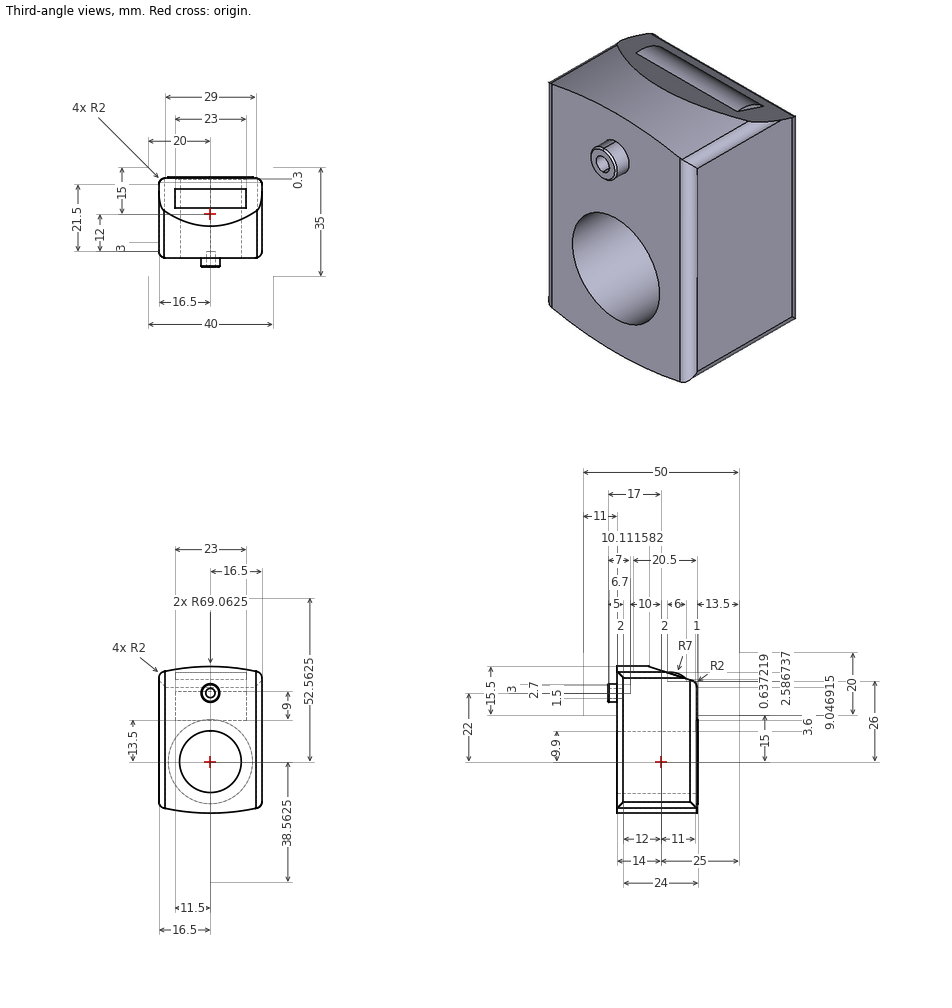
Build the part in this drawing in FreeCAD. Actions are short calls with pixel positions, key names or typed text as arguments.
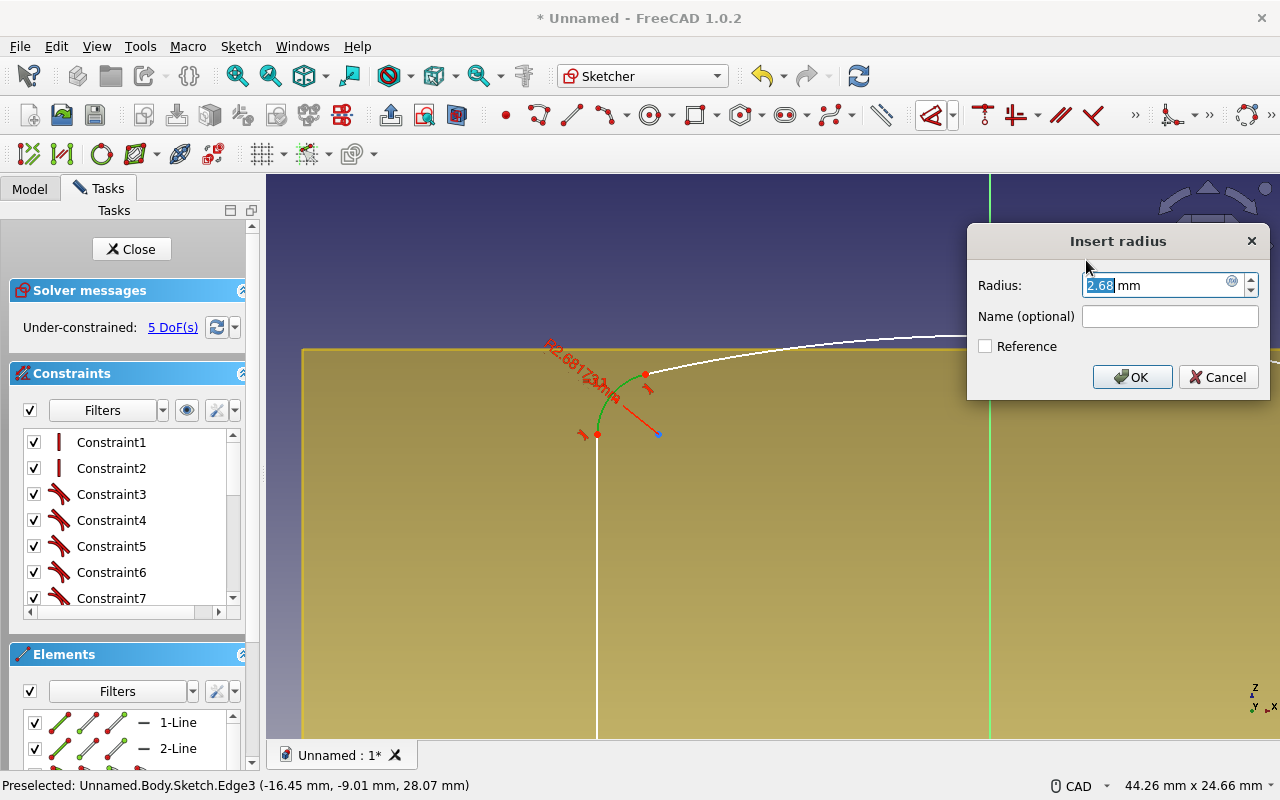
text(2)
key(Return)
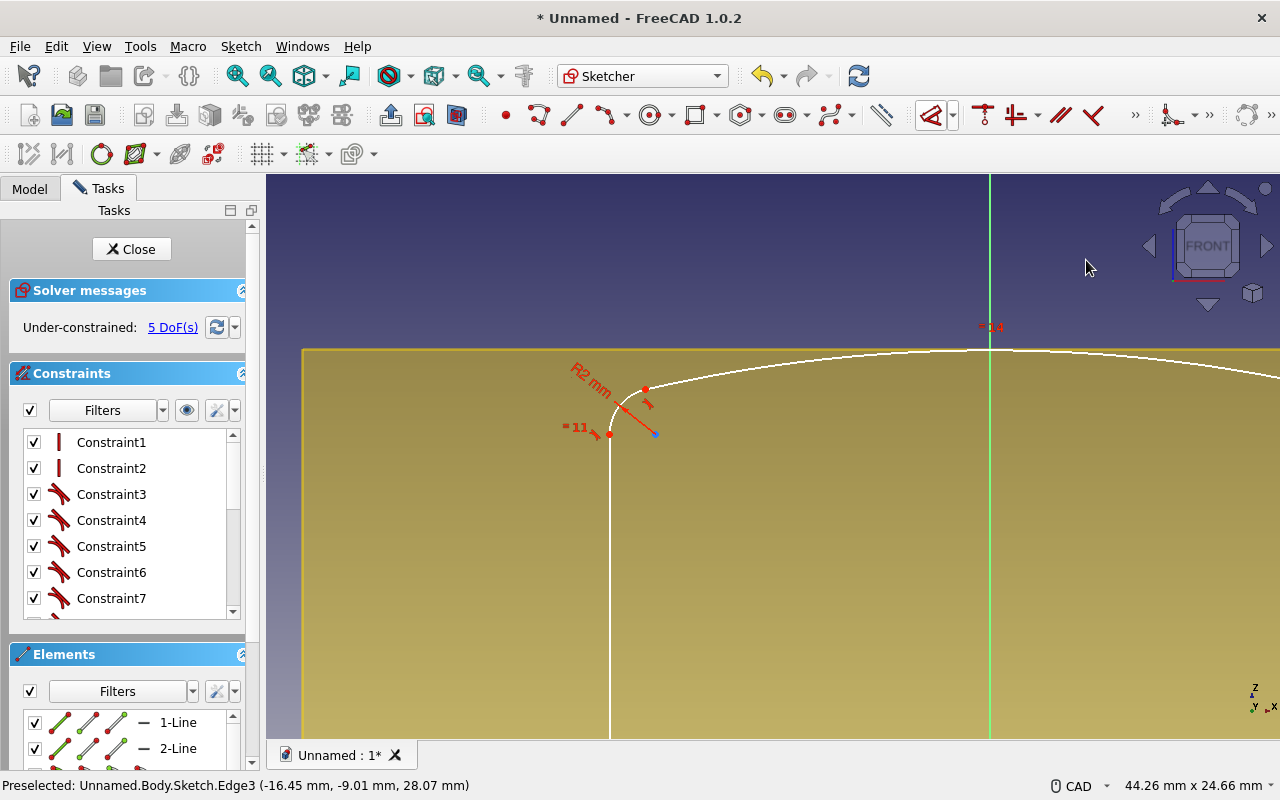
click(851, 357)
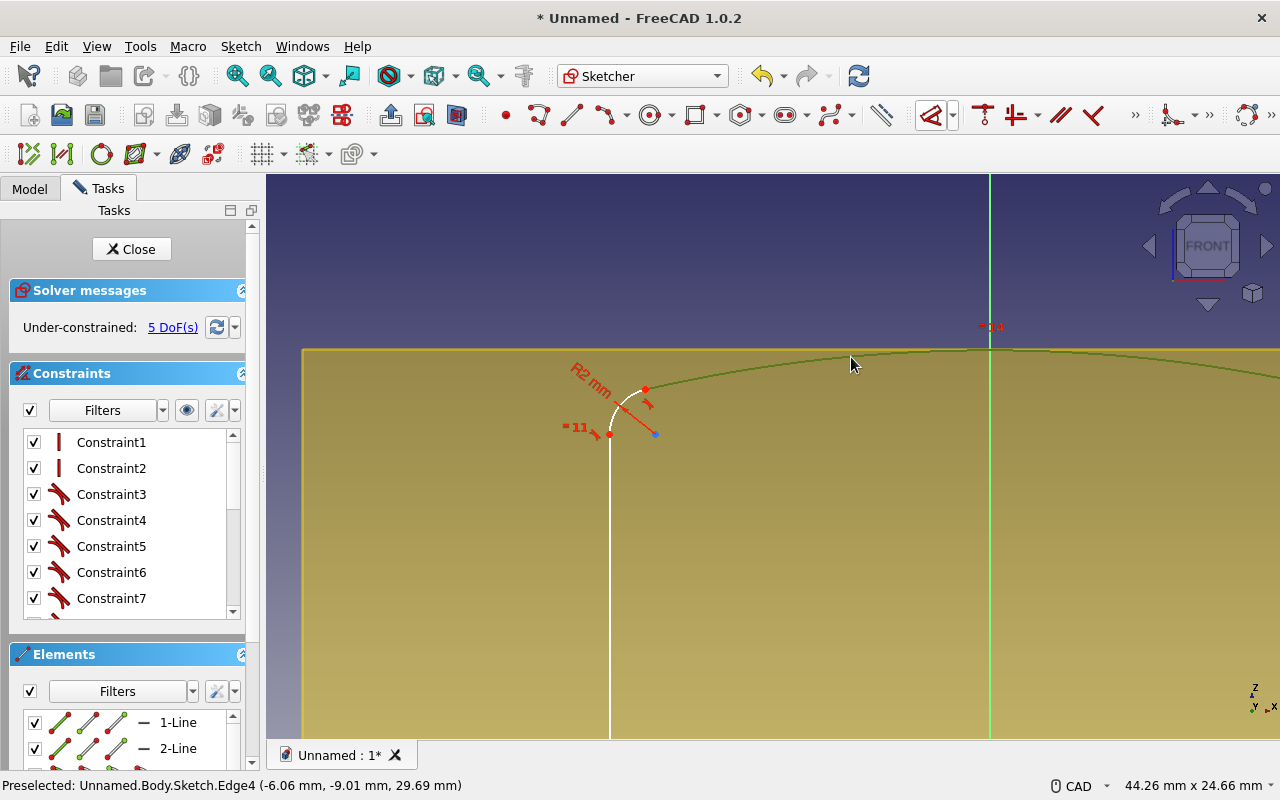
click(952, 116)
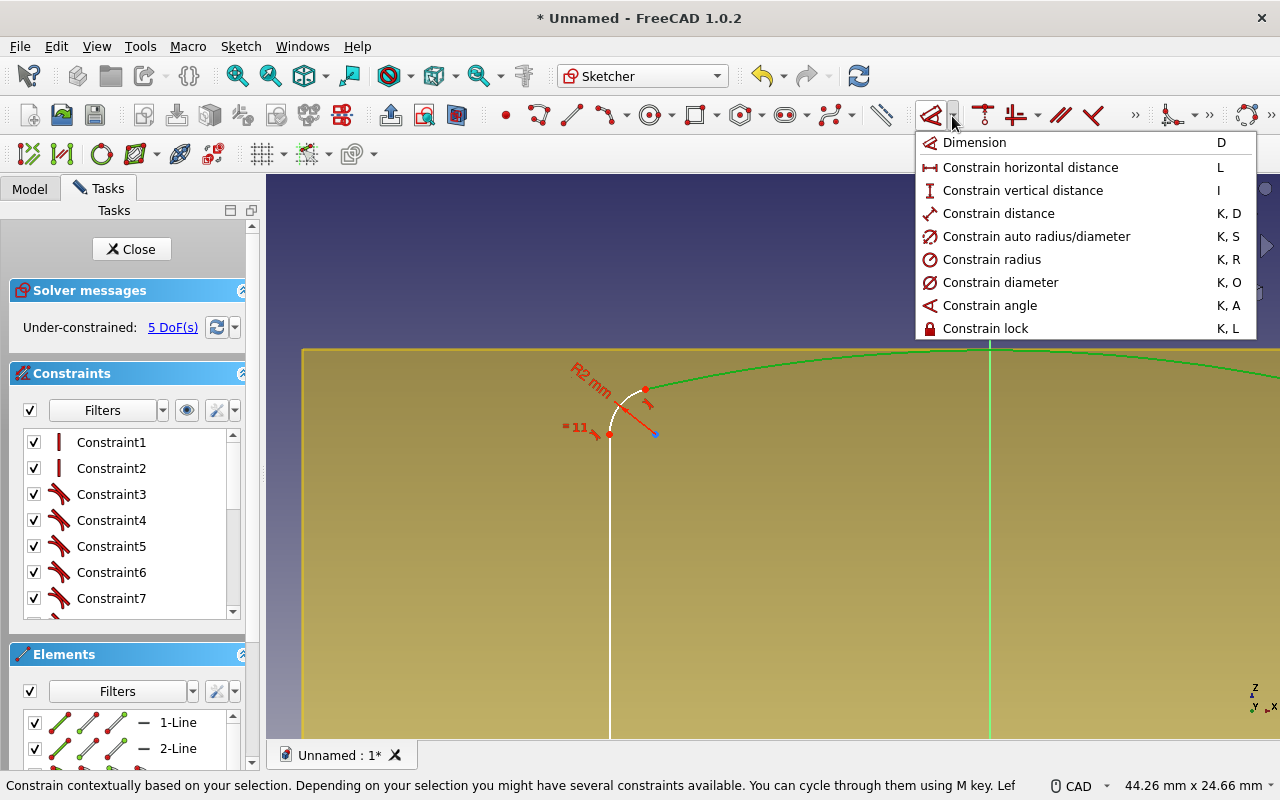
click(1086, 260)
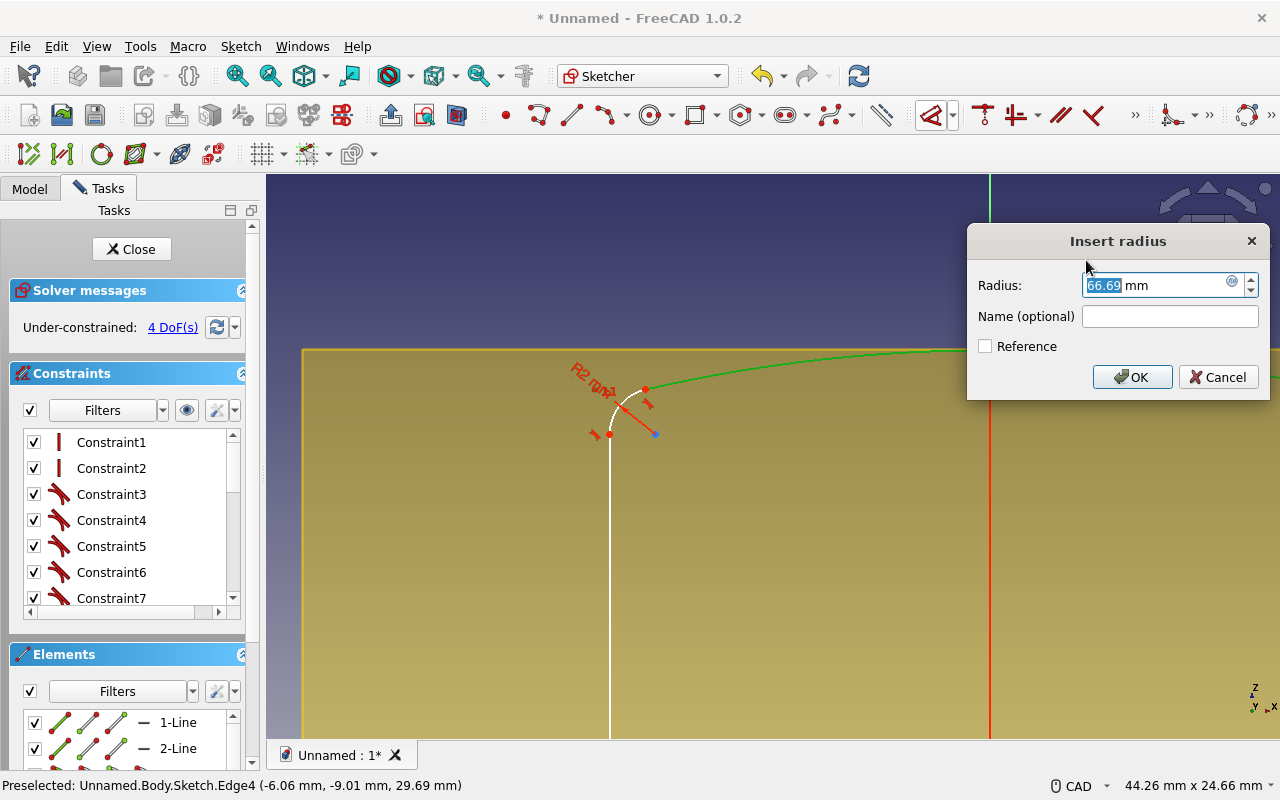
text(69.0625)
key(Return)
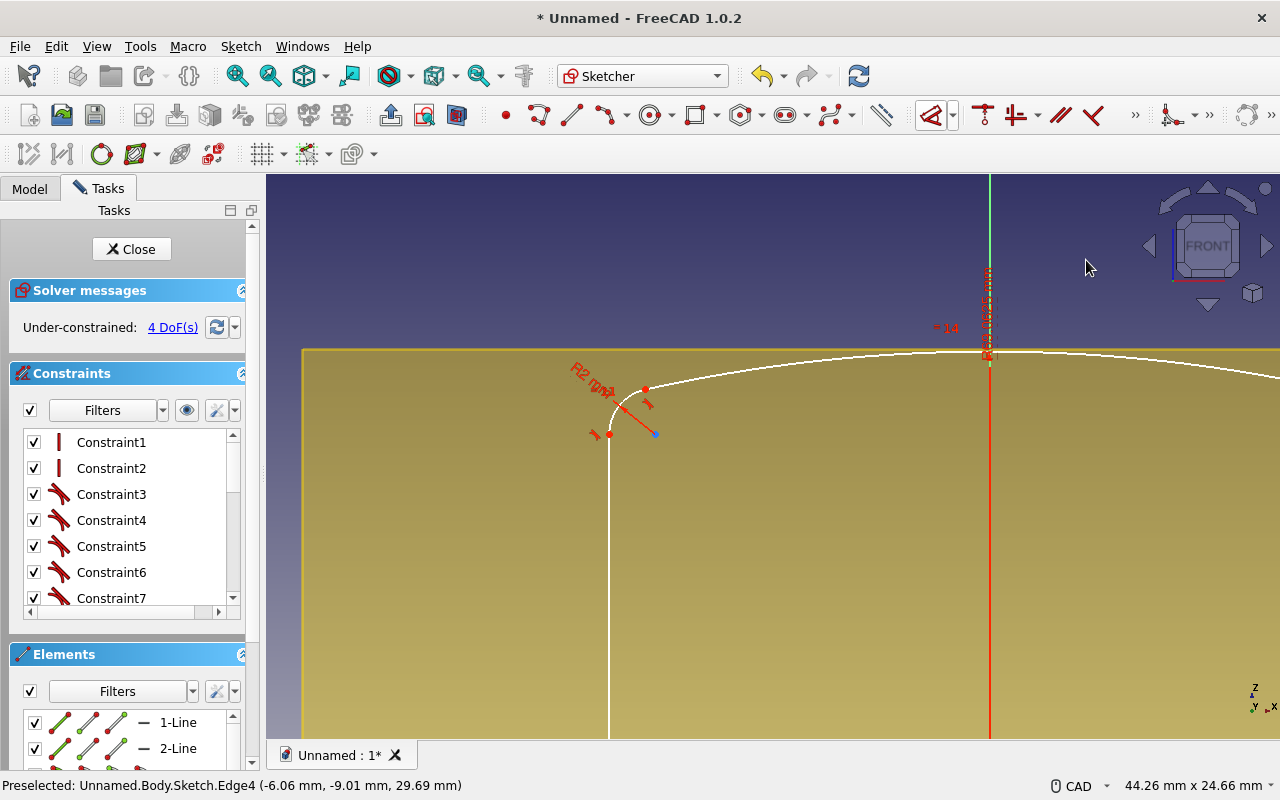
scroll(538, 212, down, 5)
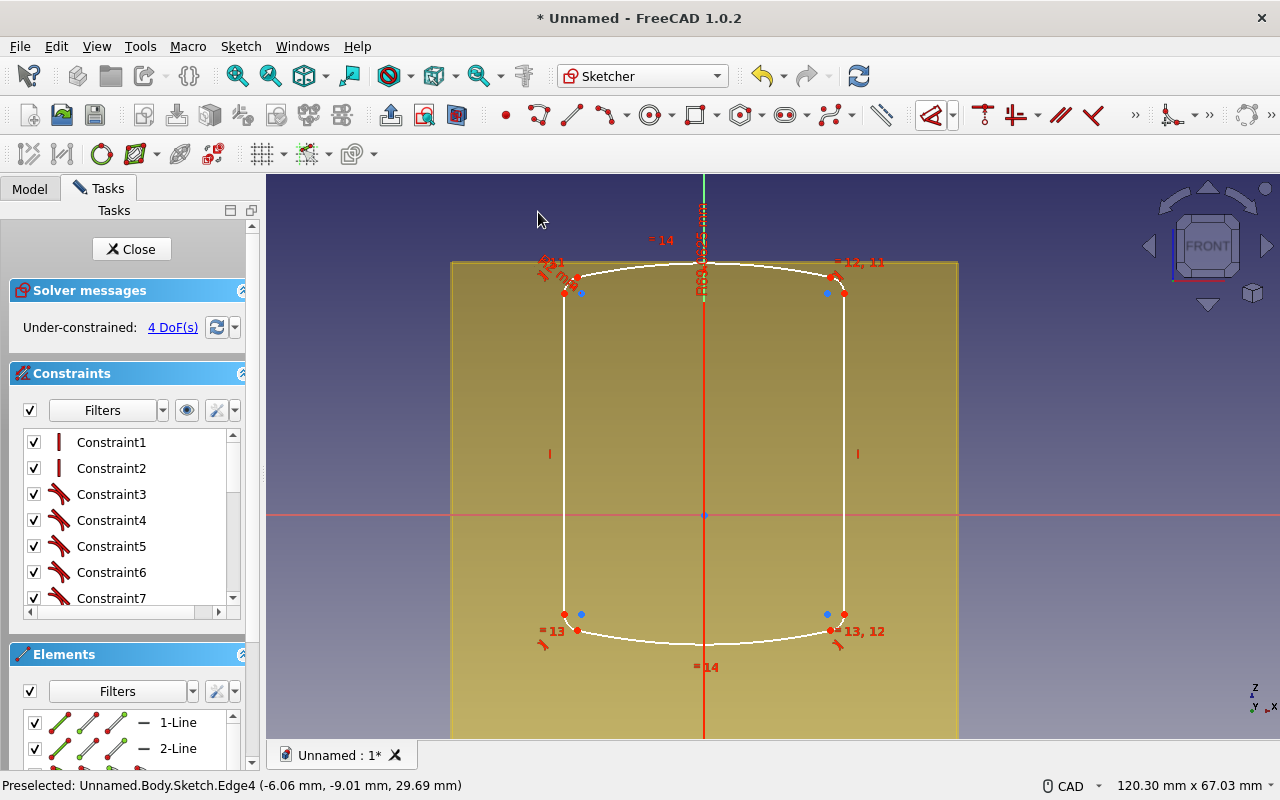
click(564, 614)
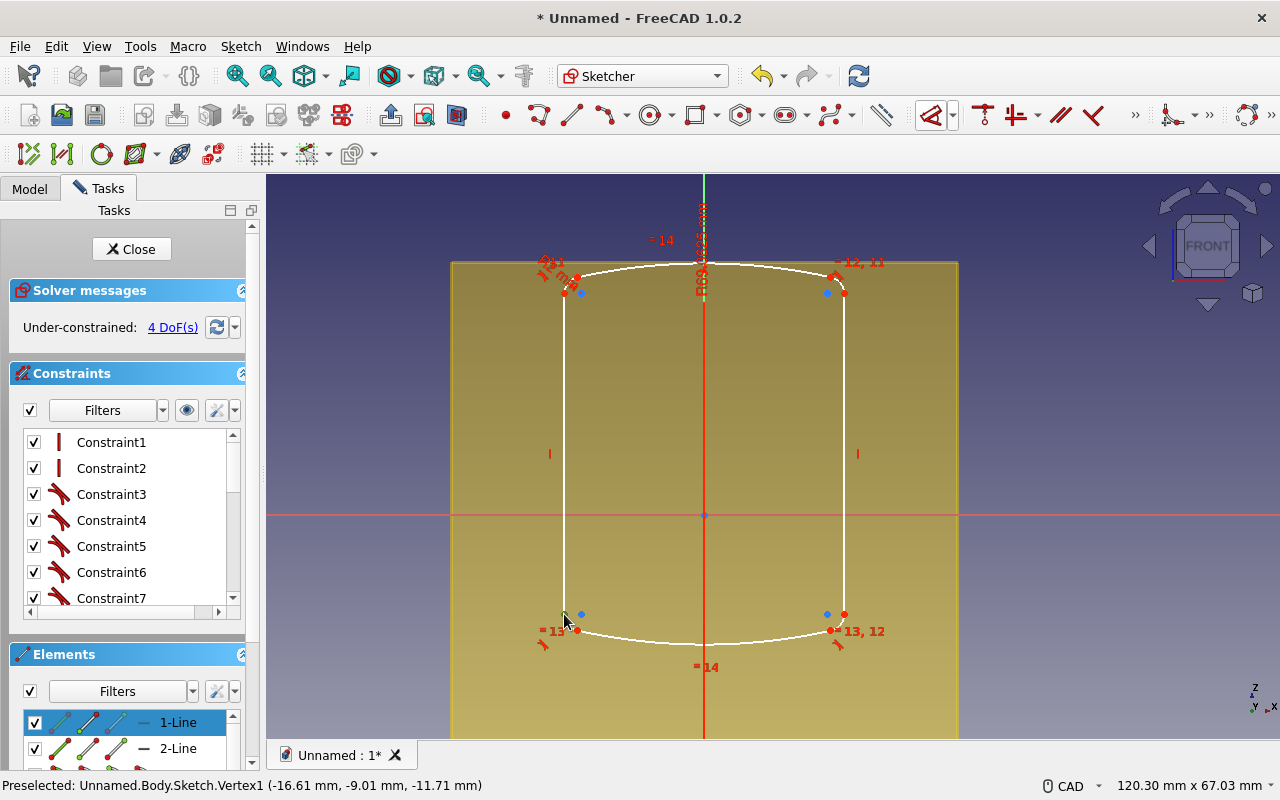
click(952, 116)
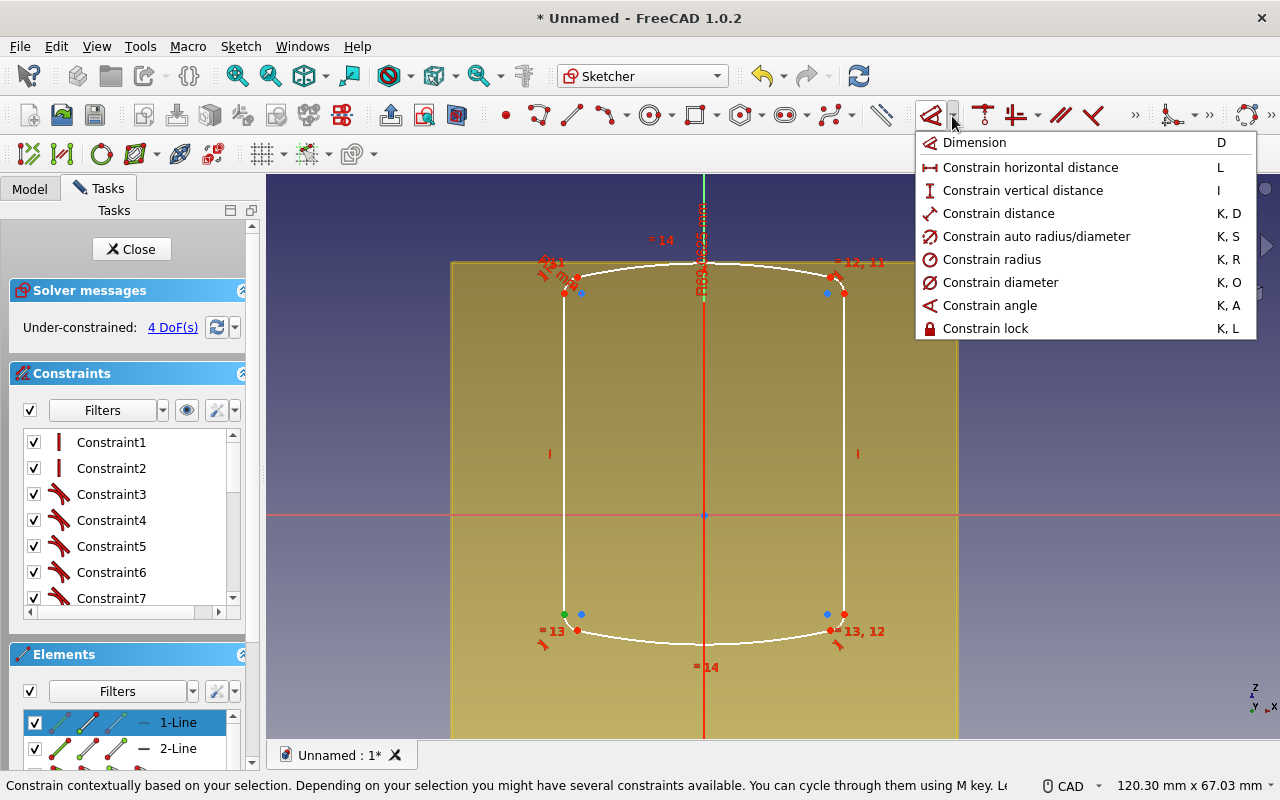
click(1086, 168)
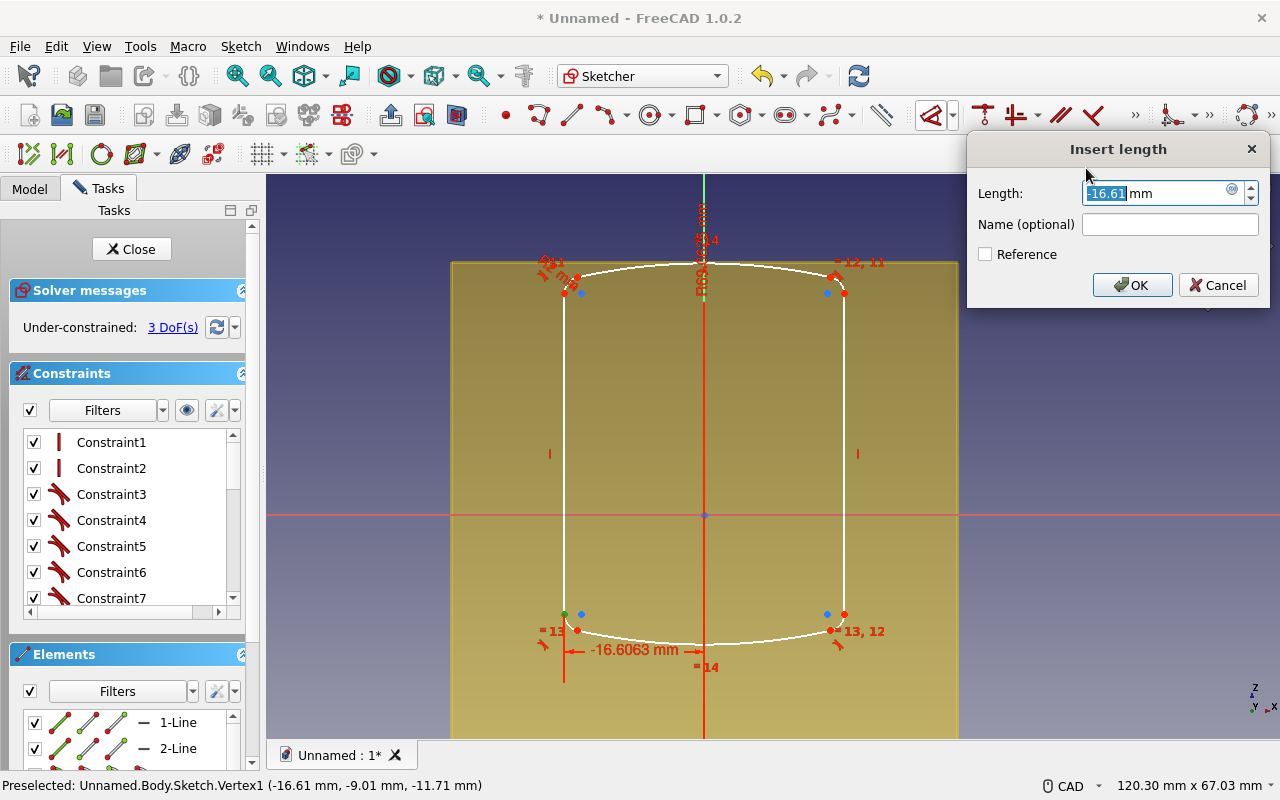
text(-16.5)
key(Return)